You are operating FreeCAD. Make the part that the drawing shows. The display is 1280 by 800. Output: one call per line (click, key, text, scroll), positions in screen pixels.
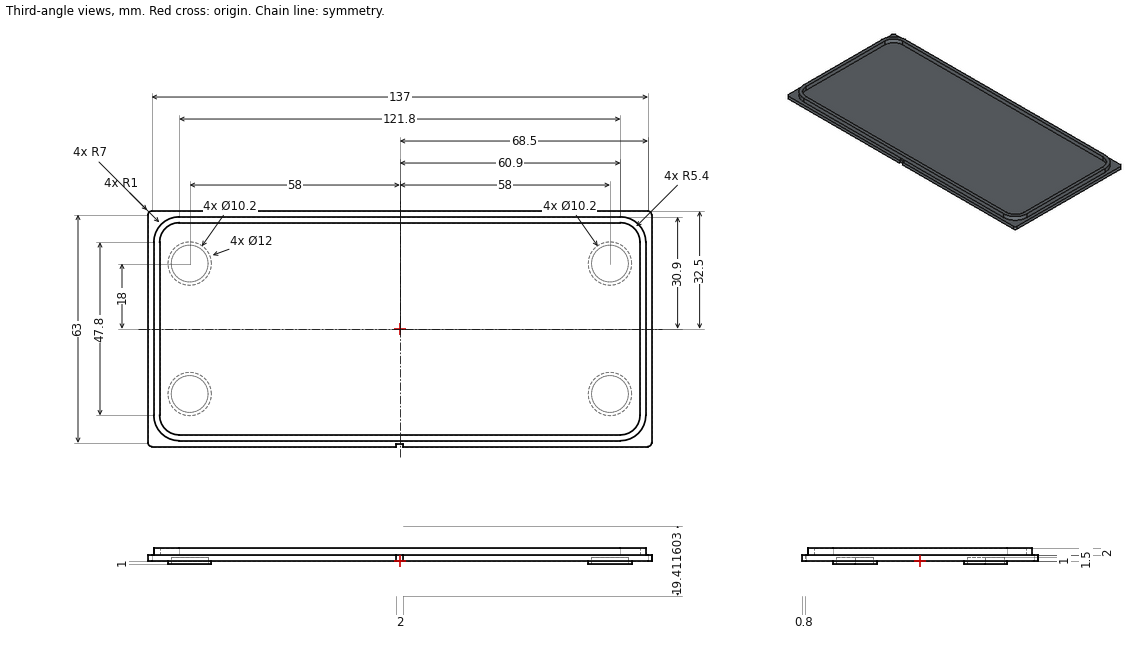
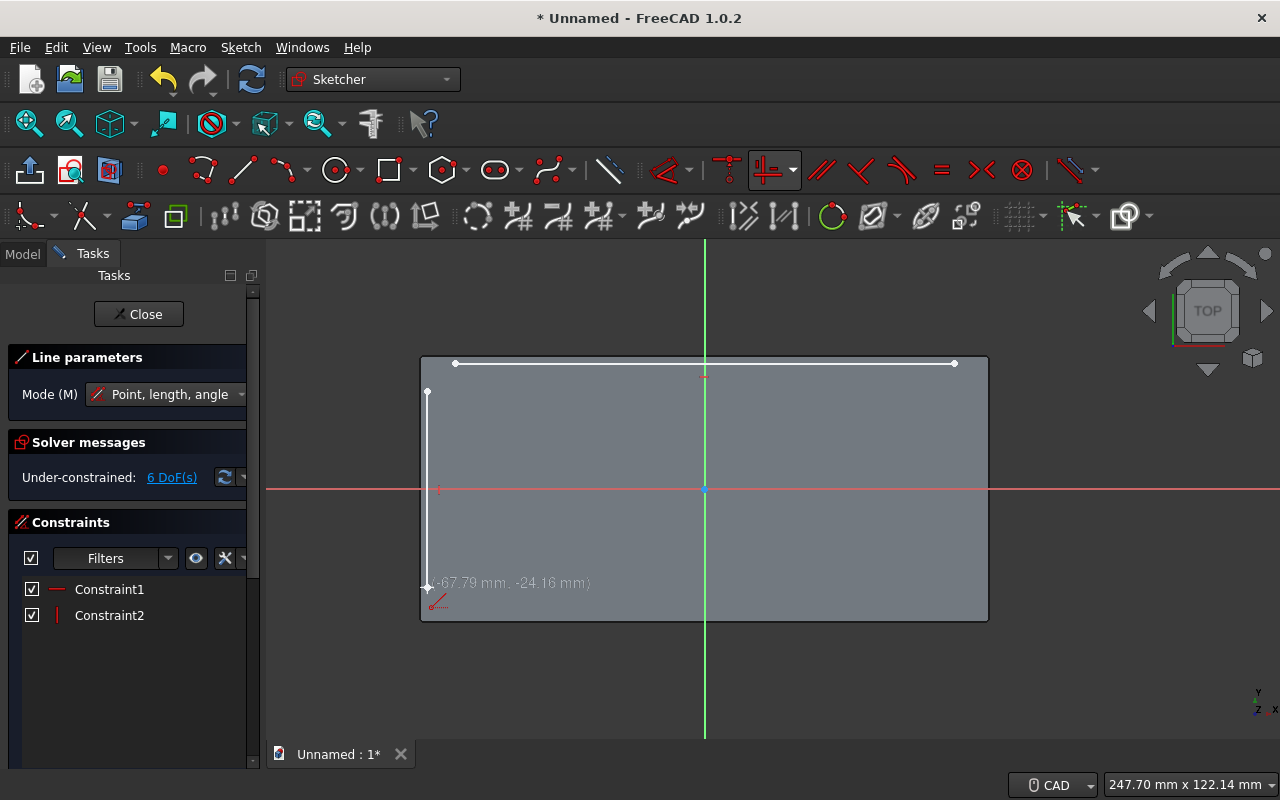
click(455, 616)
click(954, 616)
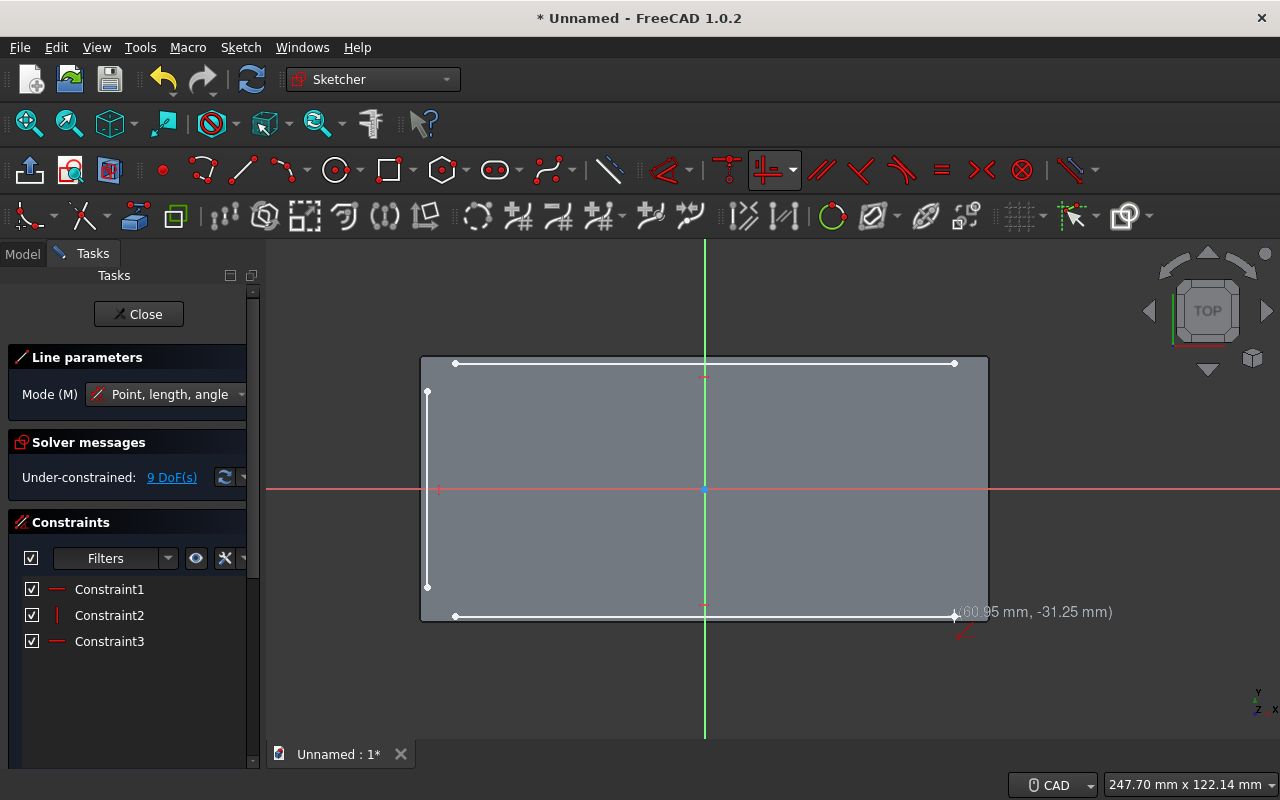
click(982, 587)
click(982, 391)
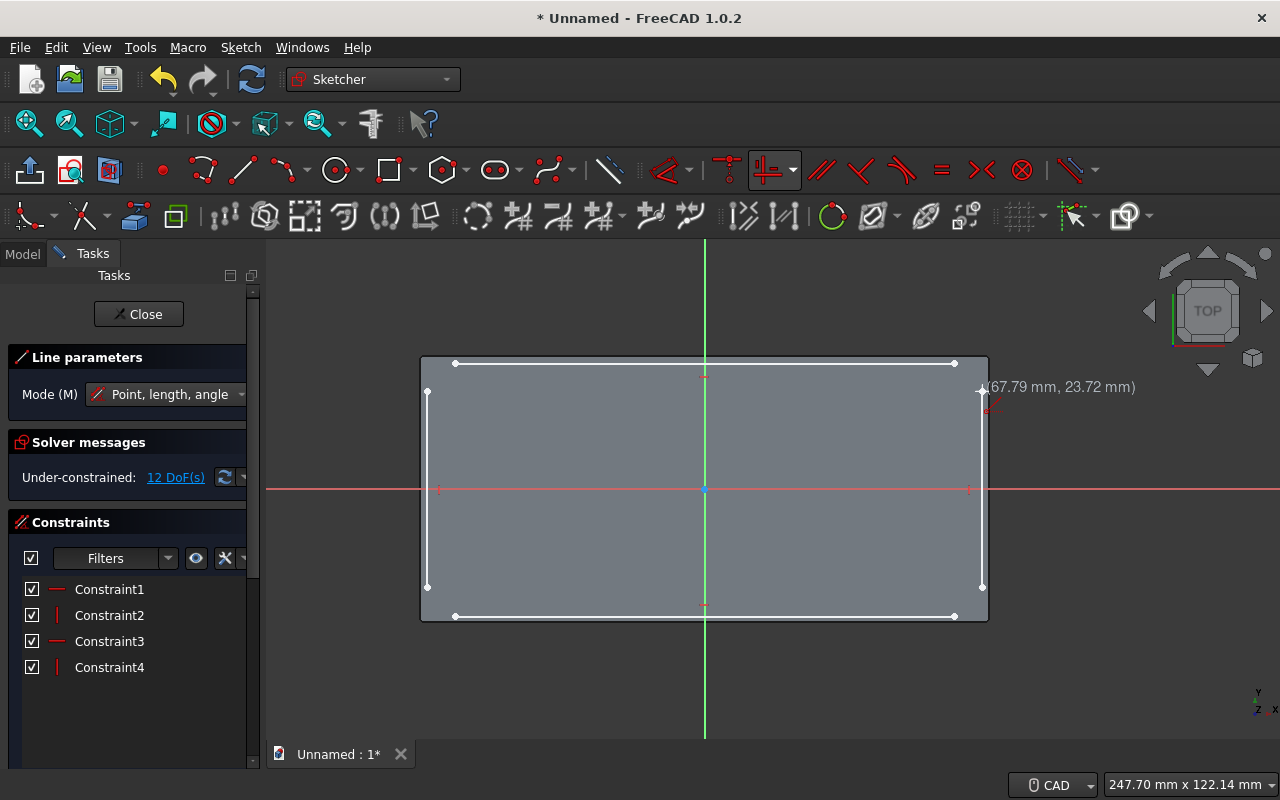
click(284, 170)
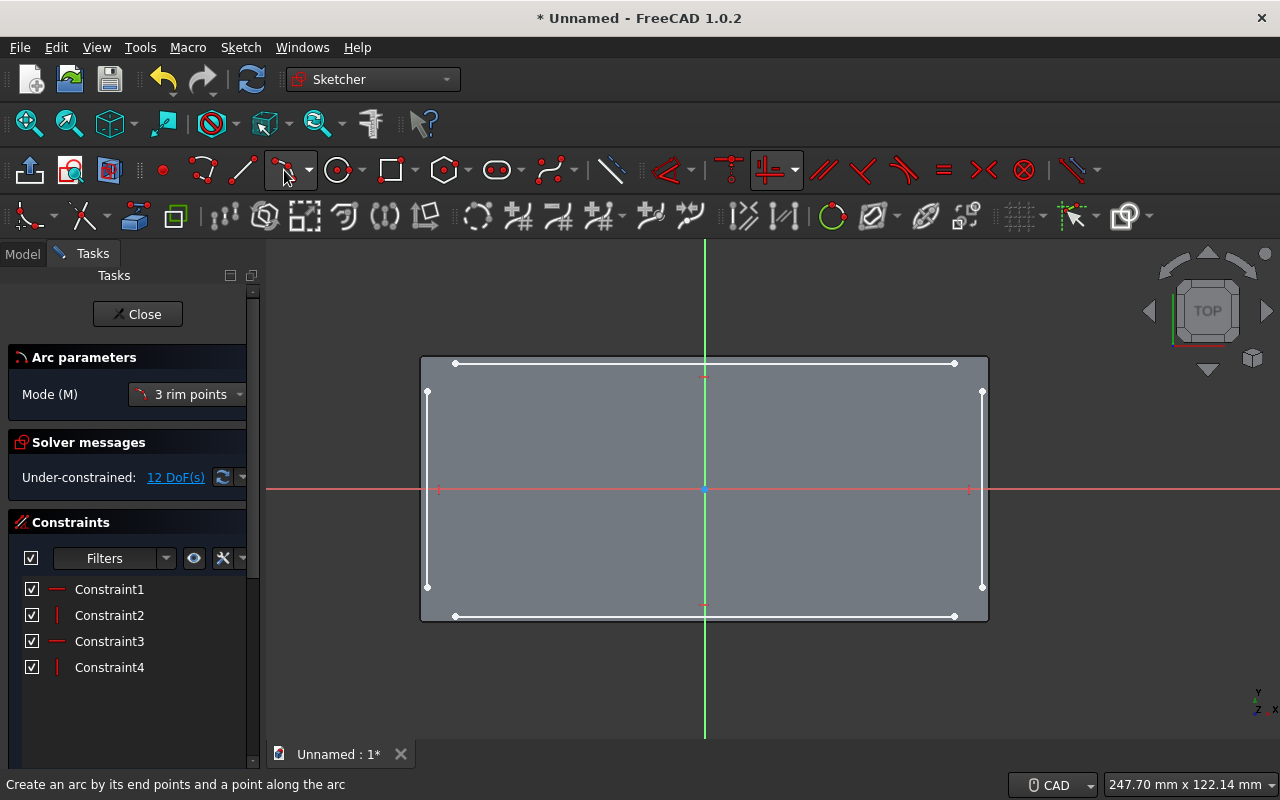
click(455, 364)
click(427, 392)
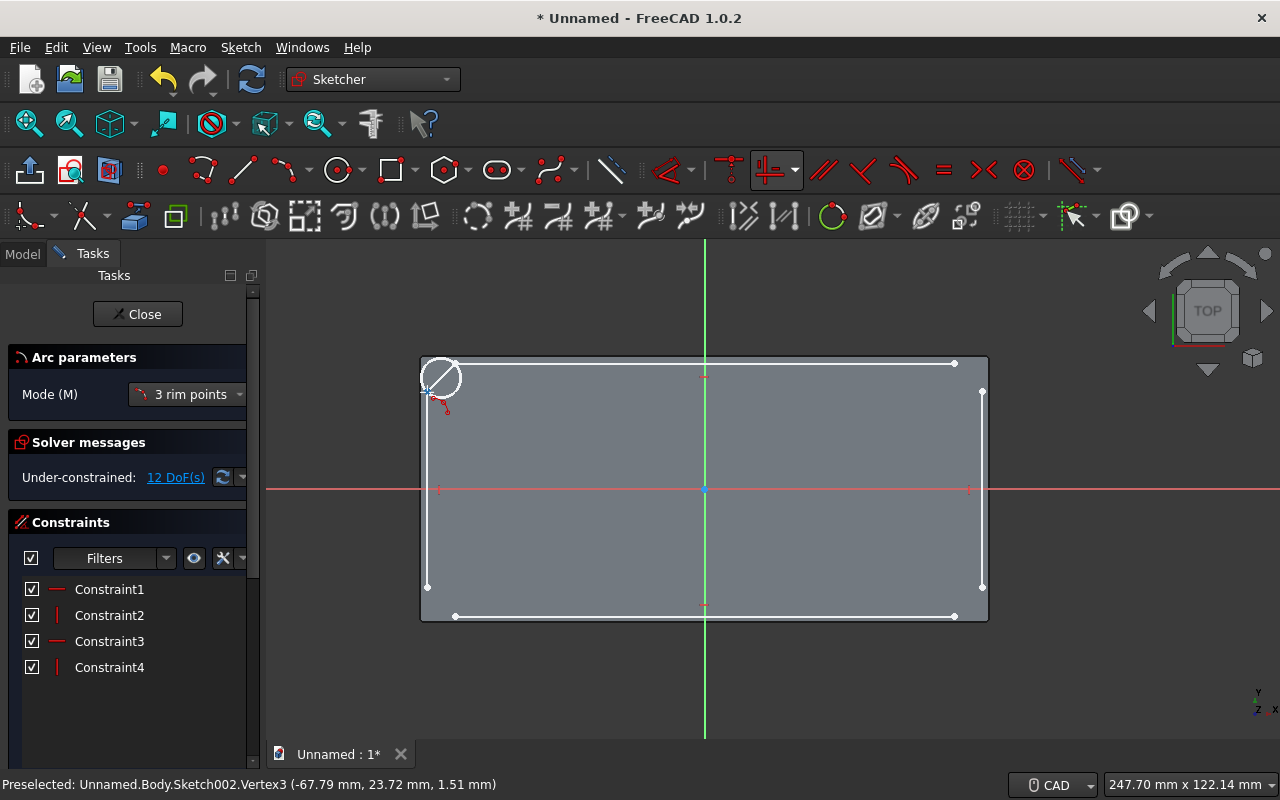
scroll(435, 371, up, 4)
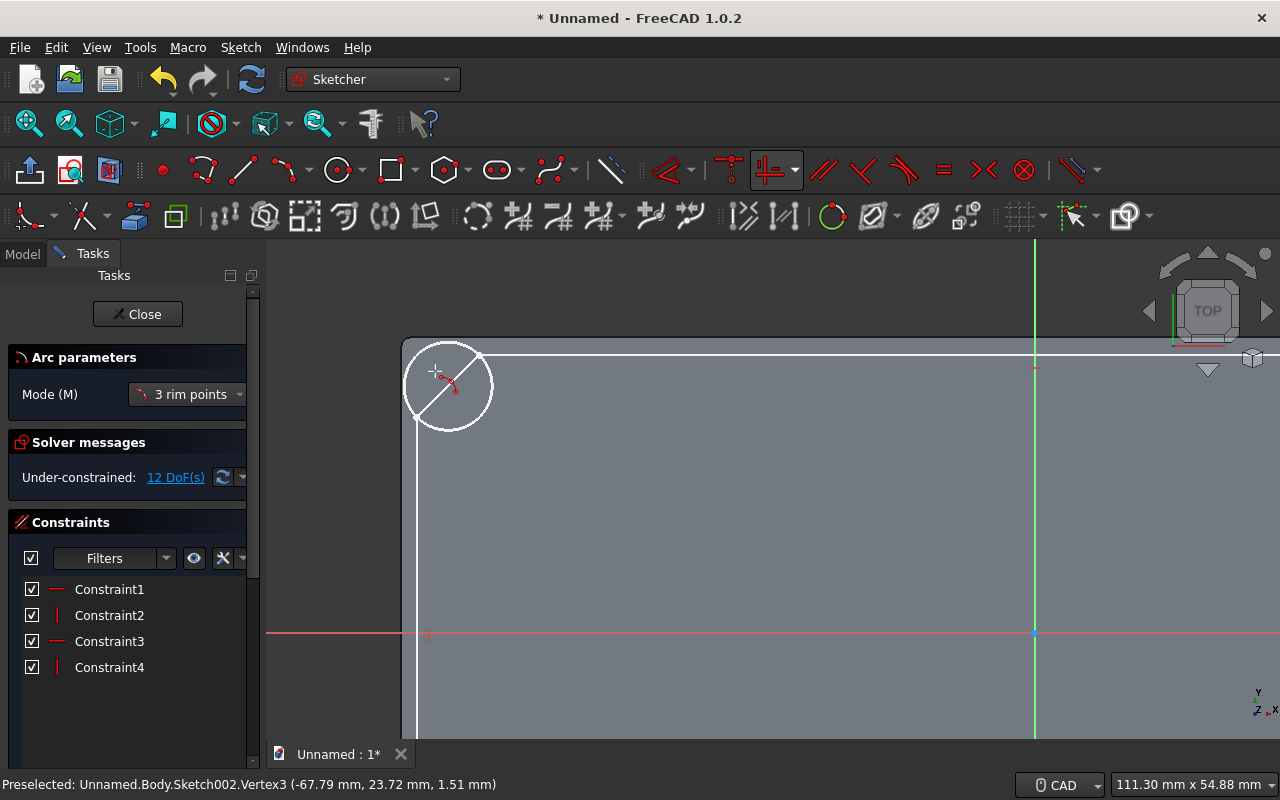
click(435, 371)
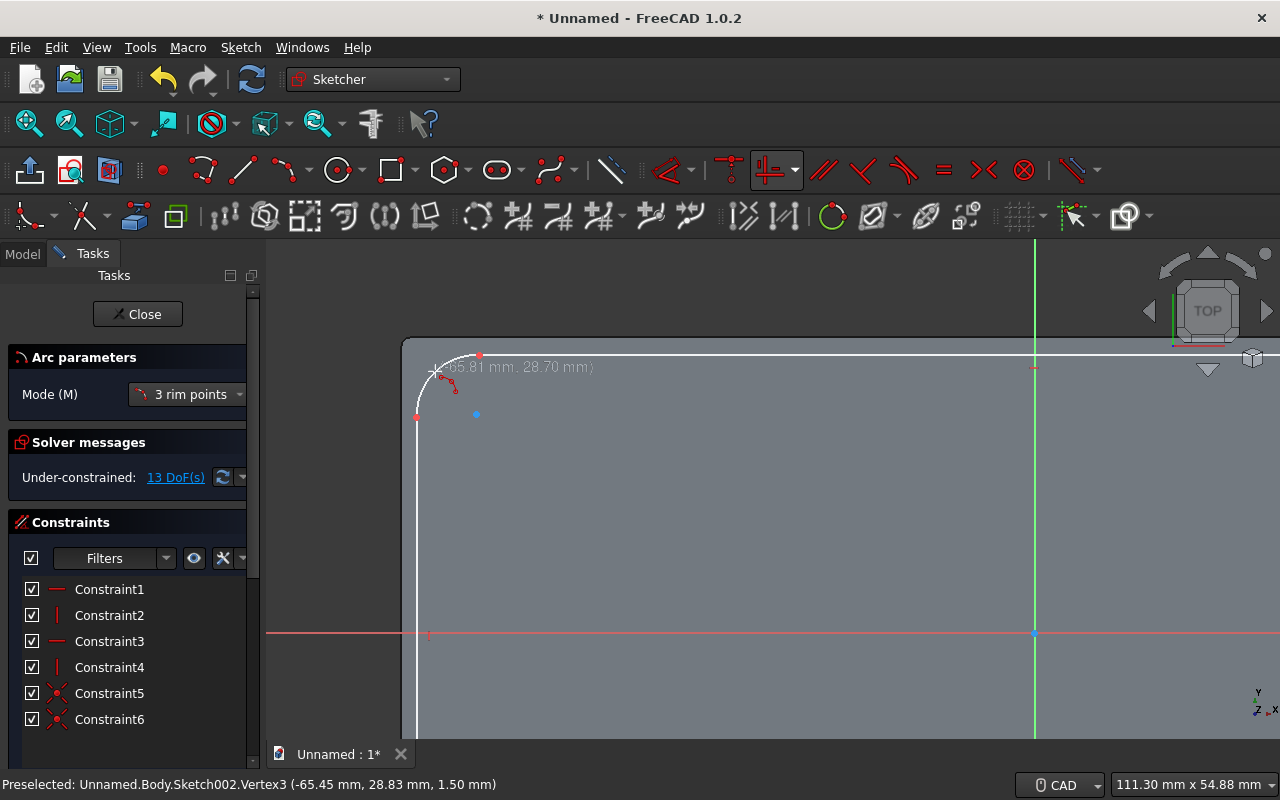
scroll(435, 371, down, 4)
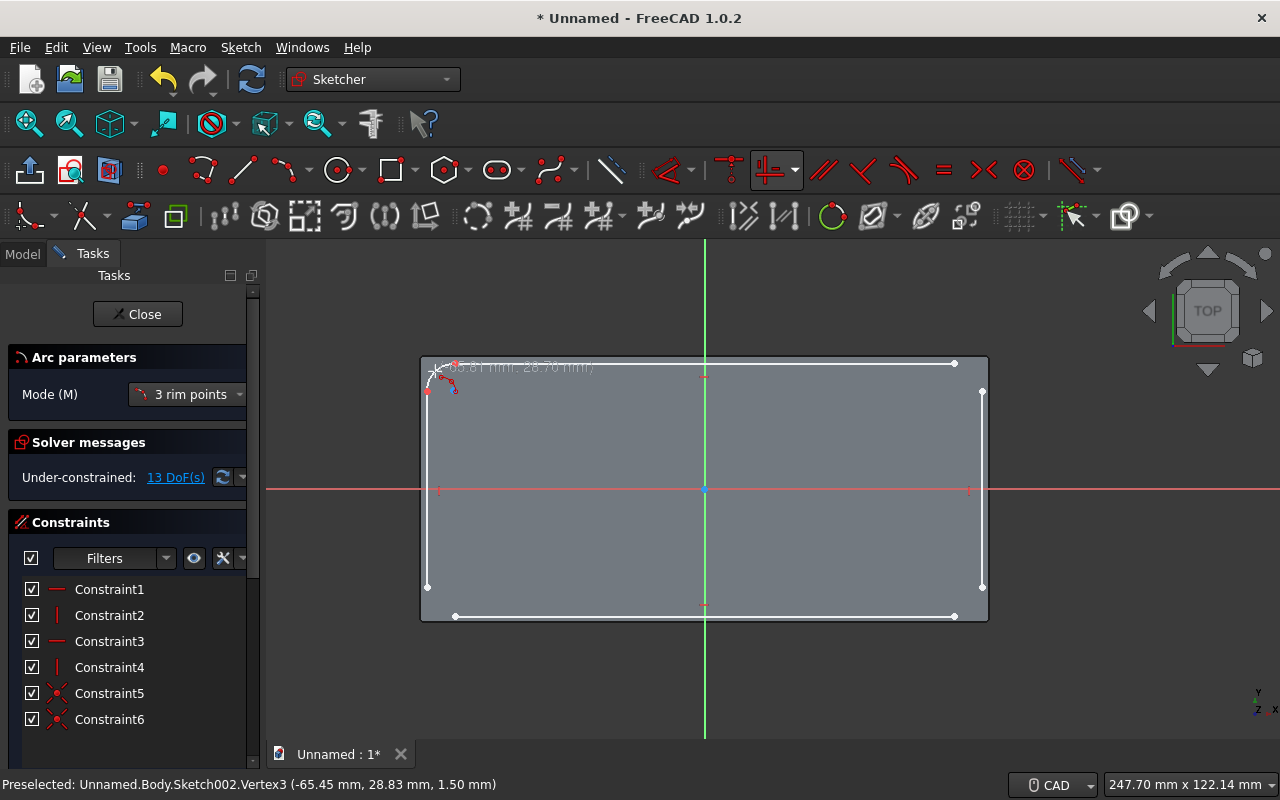
click(427, 588)
click(455, 617)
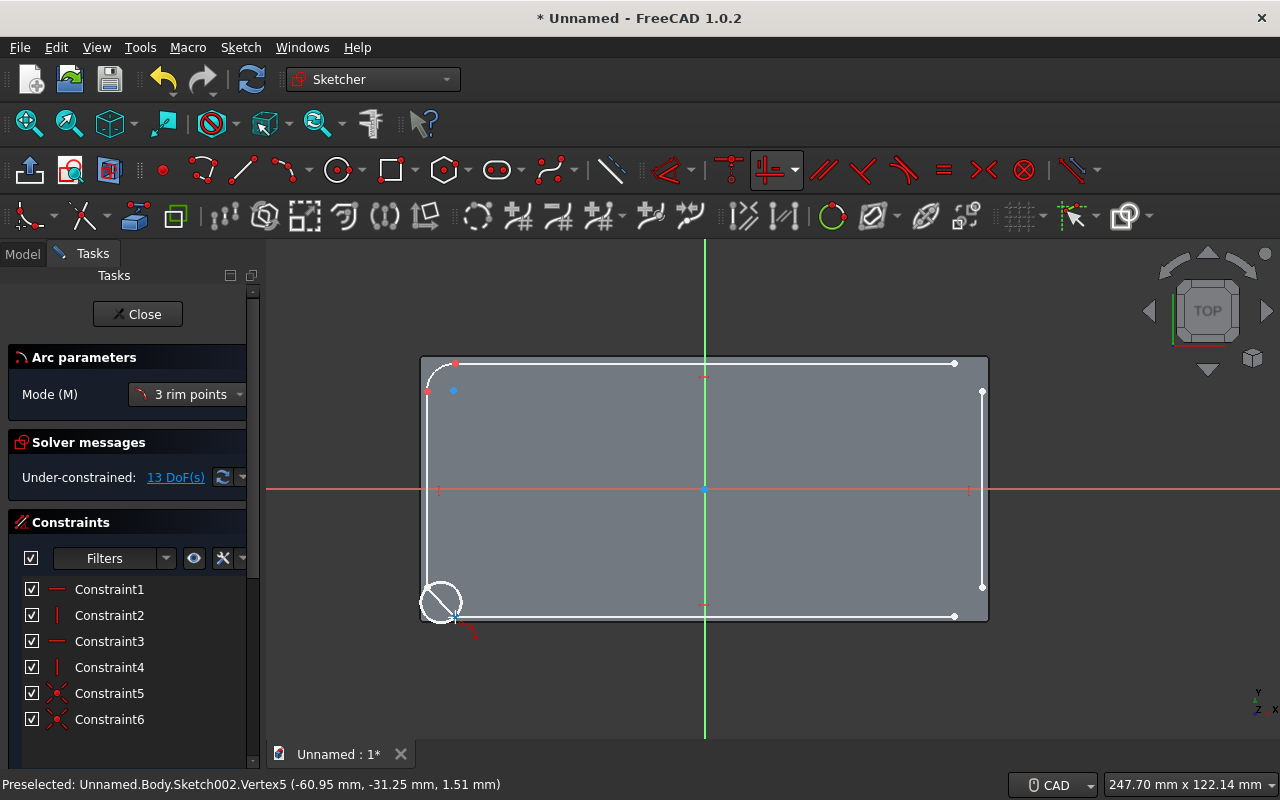
scroll(435, 607, up, 4)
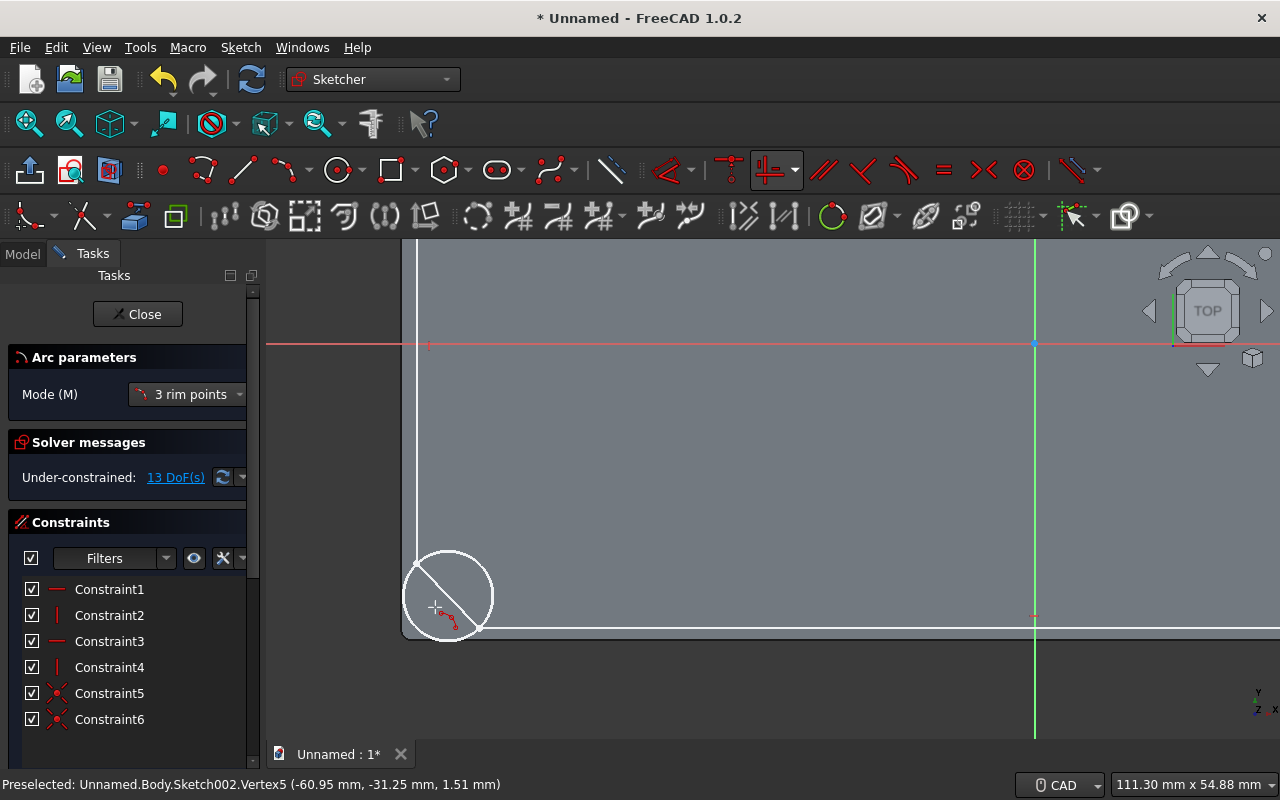
click(435, 607)